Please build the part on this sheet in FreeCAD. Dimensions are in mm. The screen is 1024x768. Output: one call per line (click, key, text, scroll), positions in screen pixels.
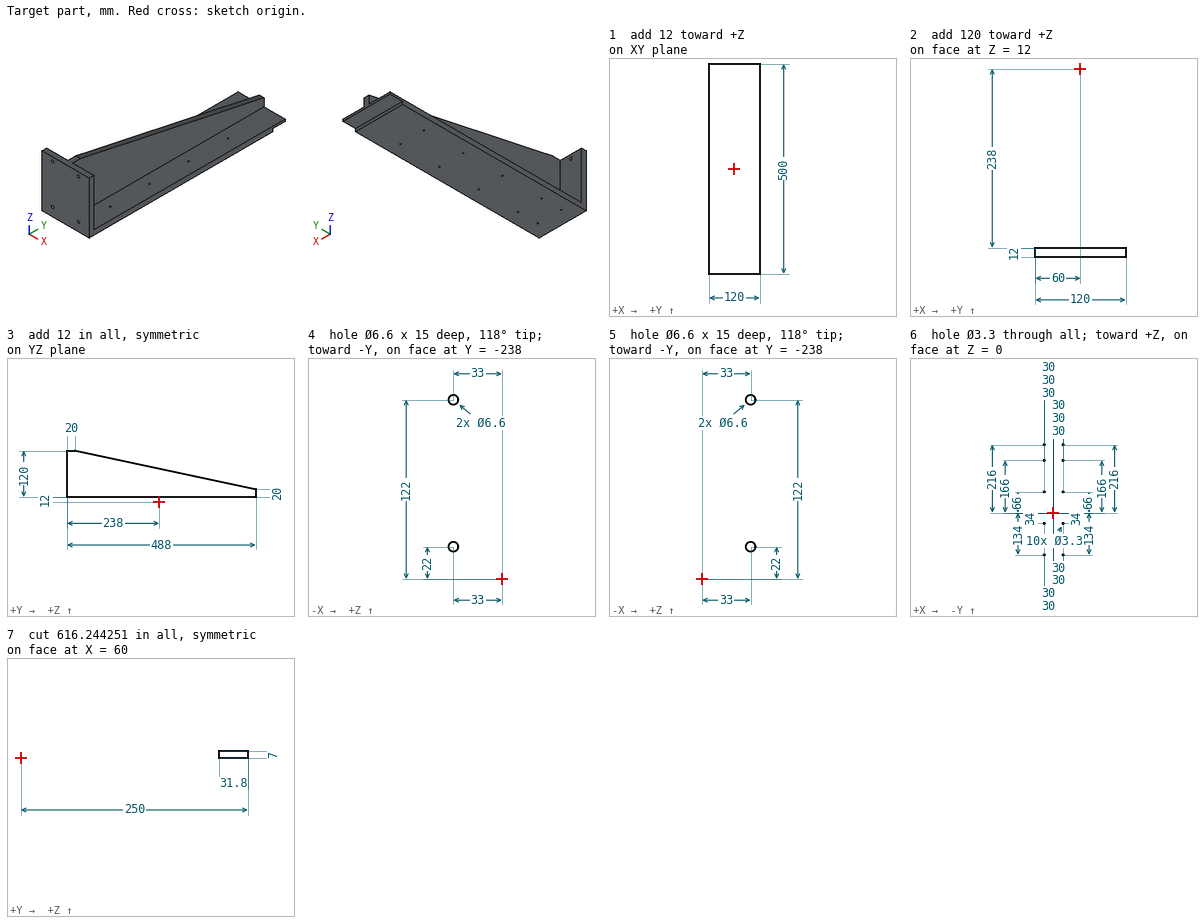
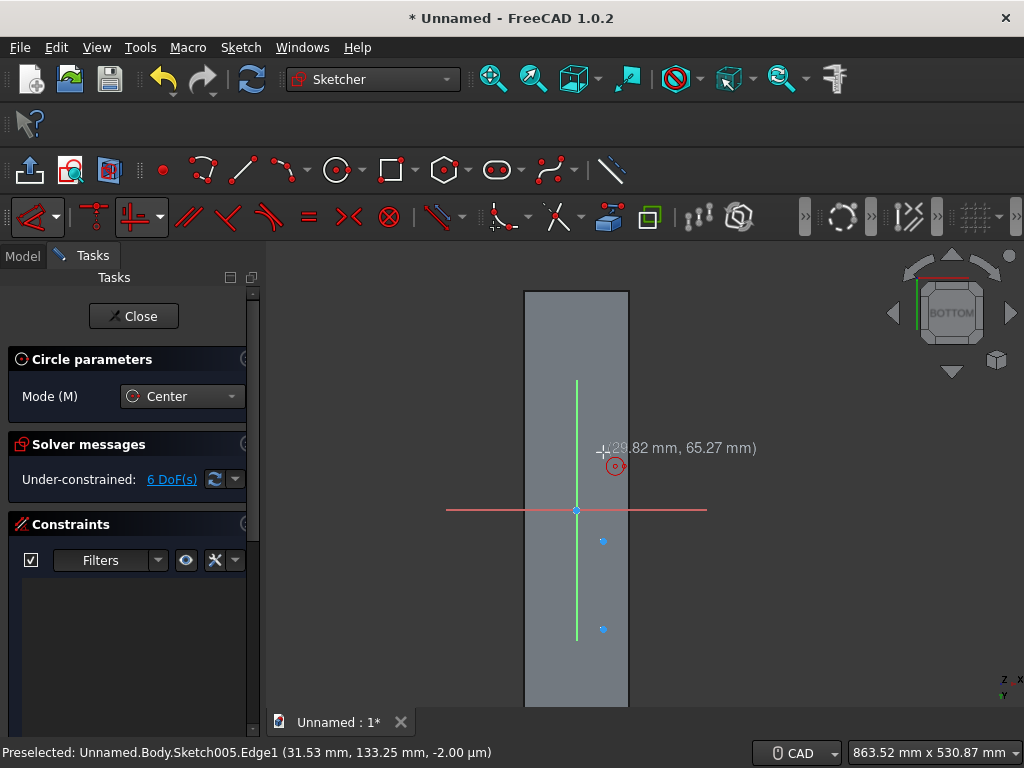
click(603, 452)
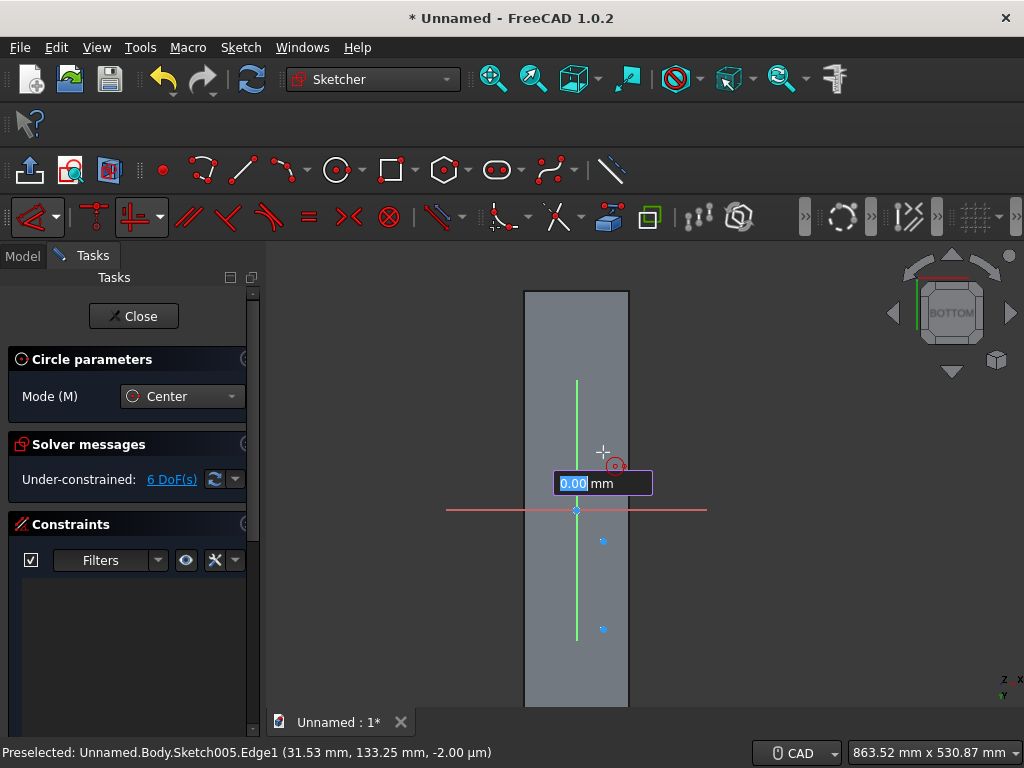
scroll(604, 451, up, 12)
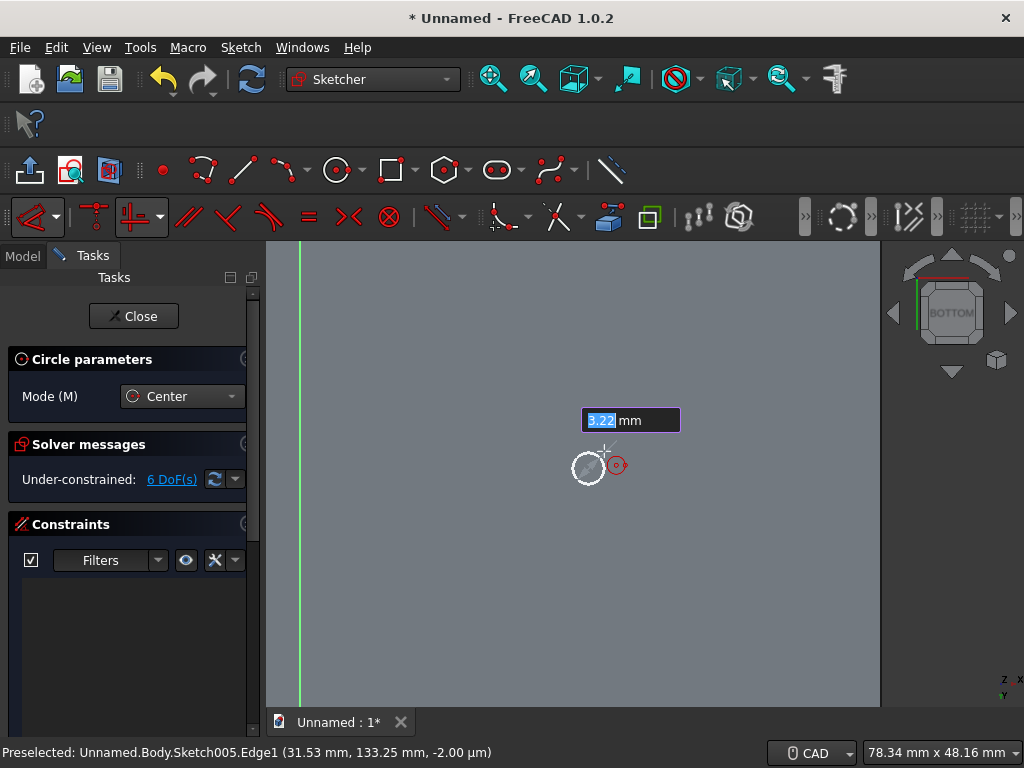
click(602, 450)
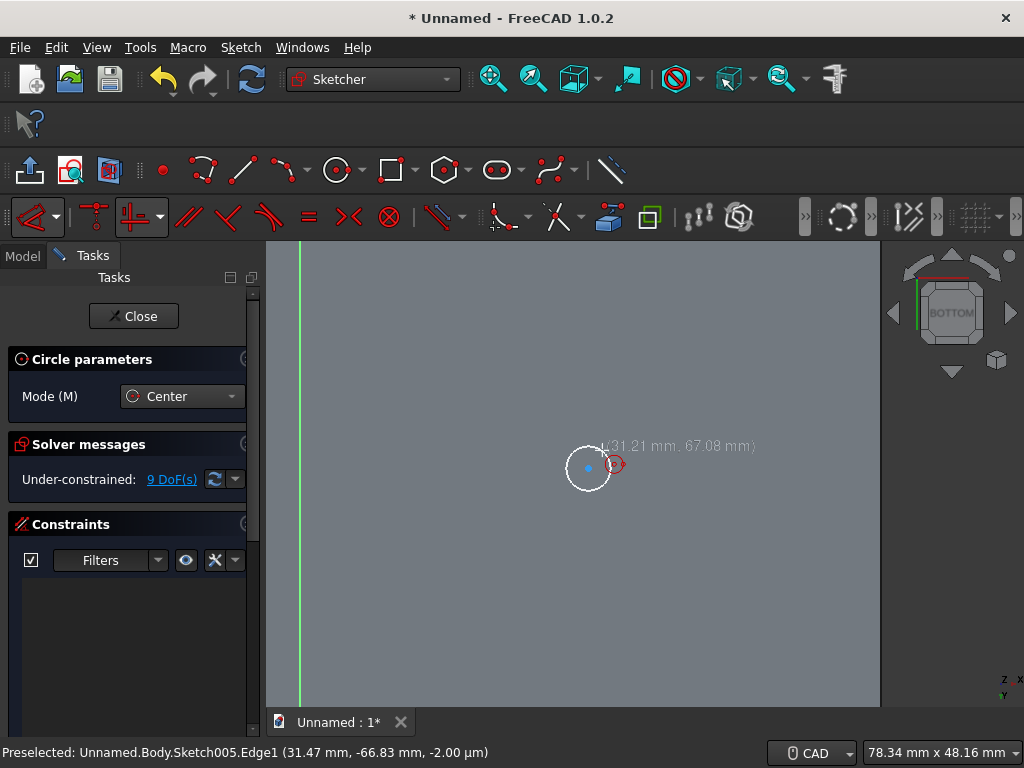
scroll(604, 451, down, 12)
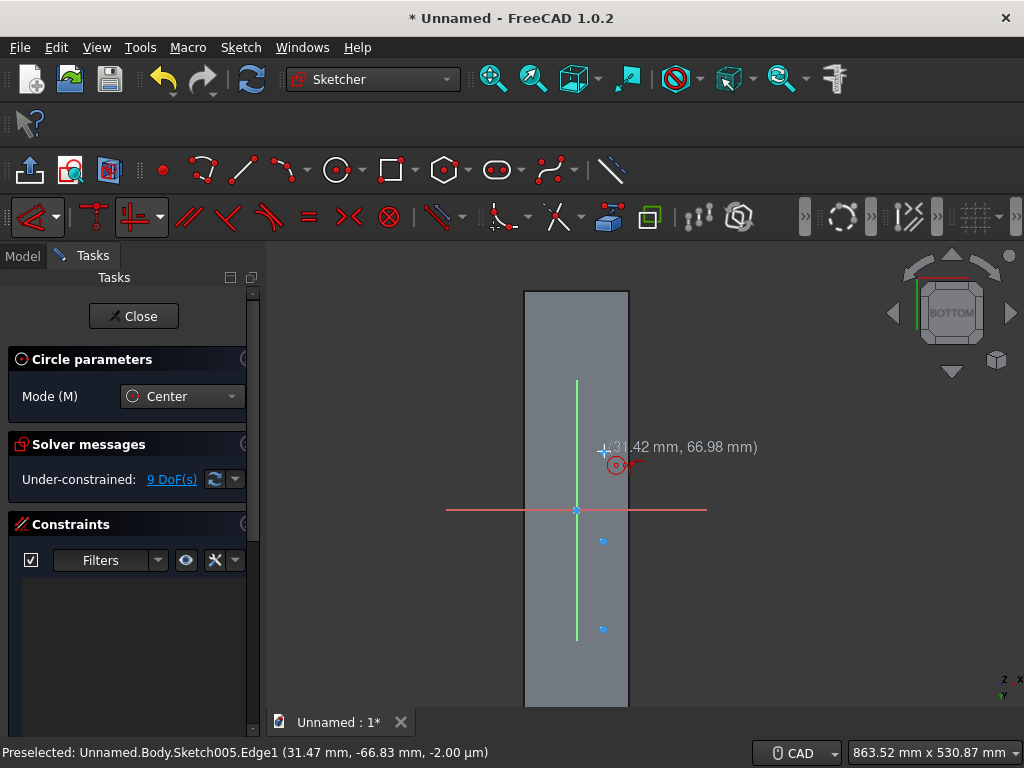
scroll(603, 365, up, 14)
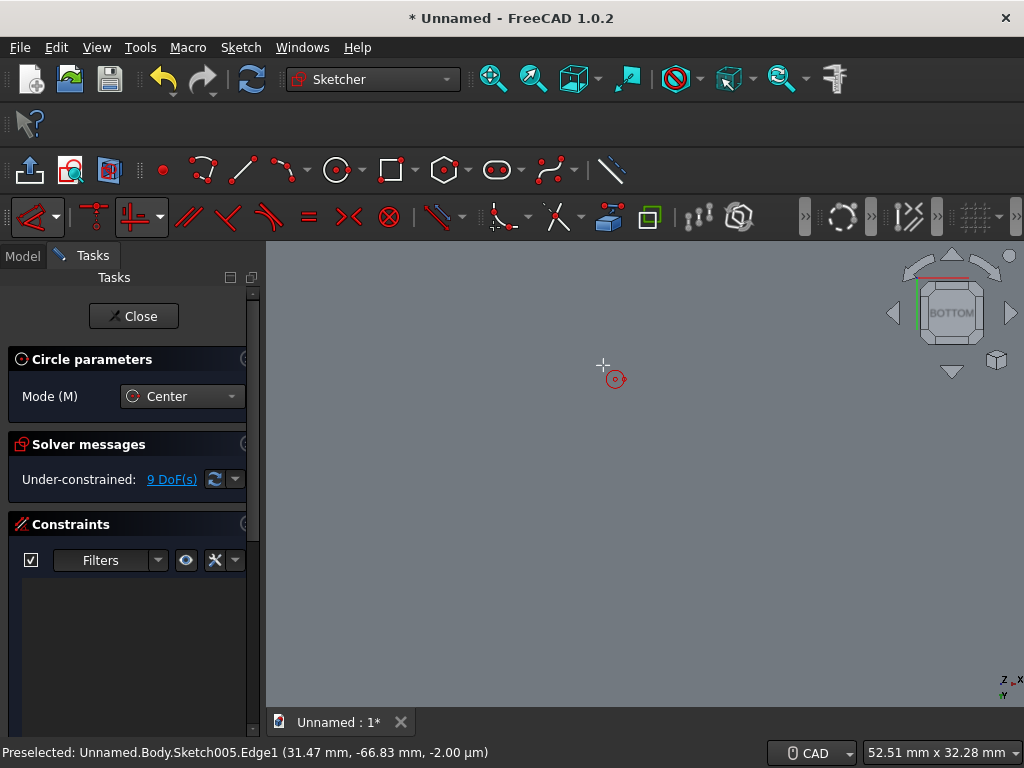
scroll(603, 365, down, 14)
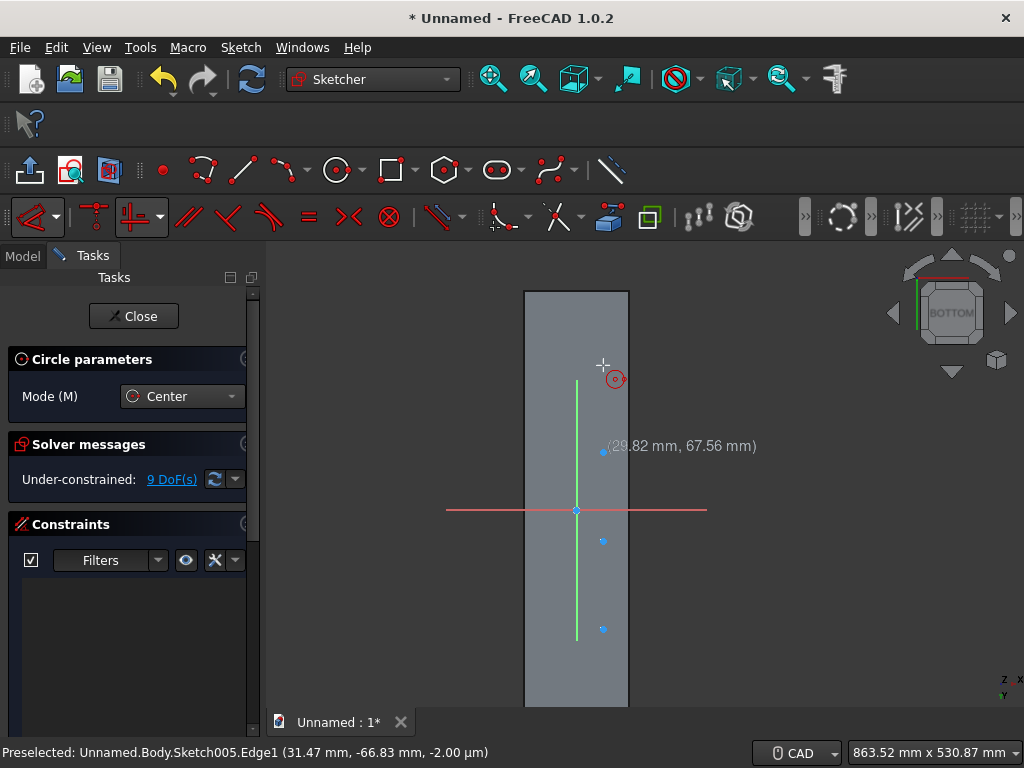
click(603, 365)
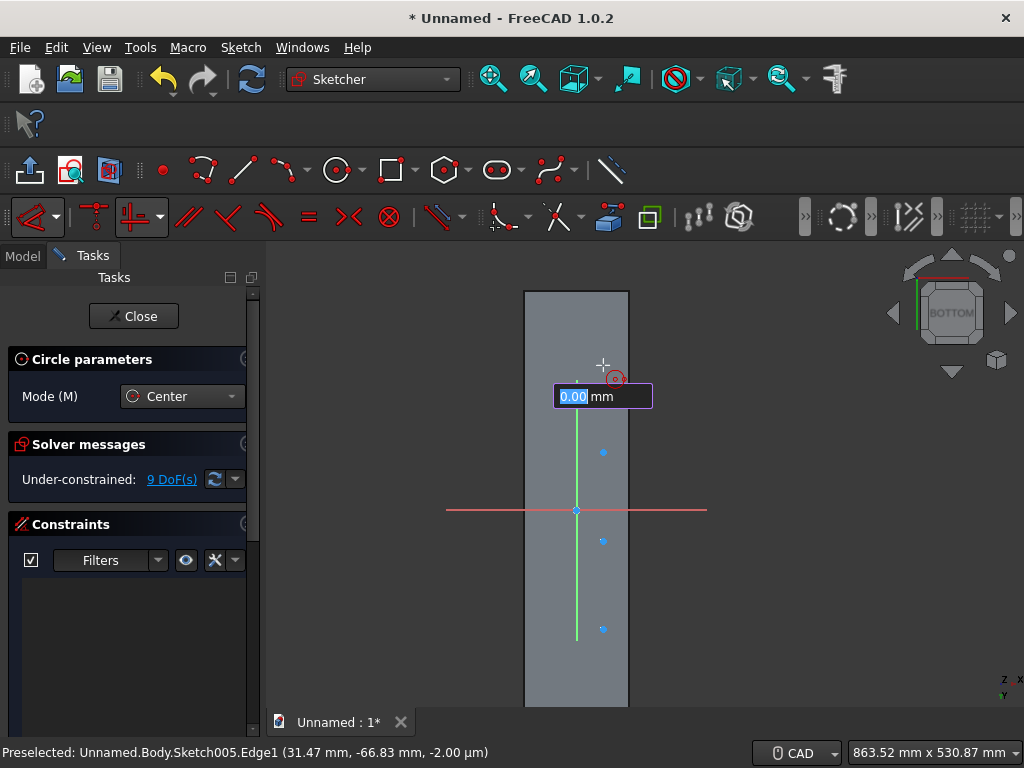
scroll(604, 364, up, 12)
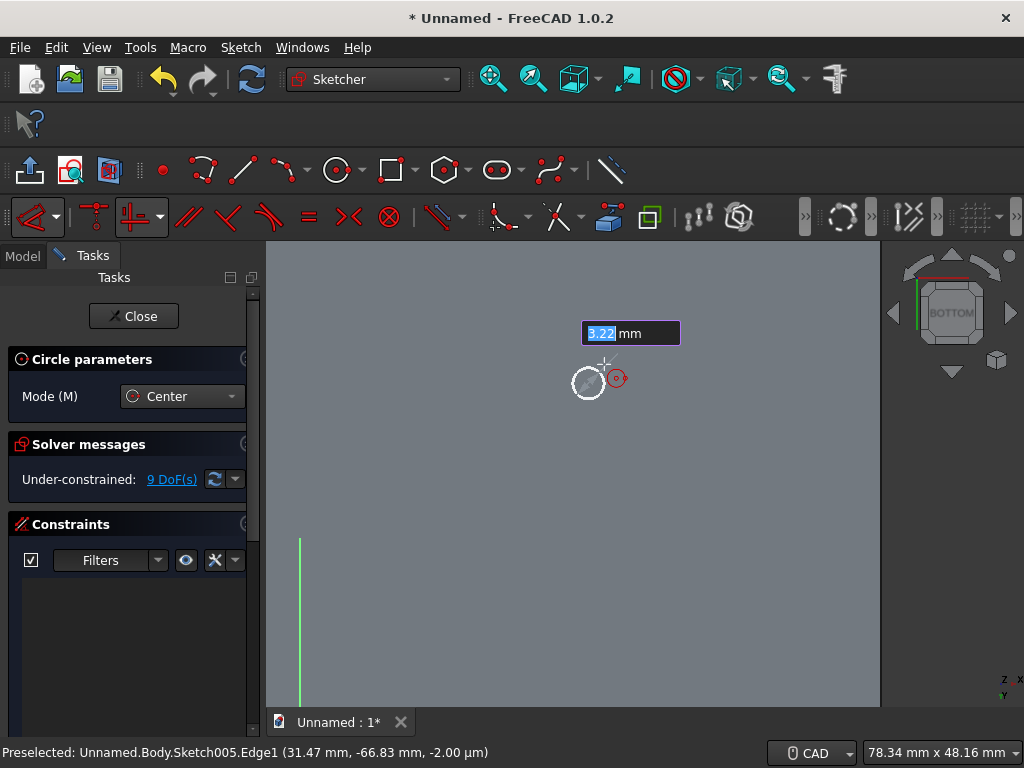
click(602, 356)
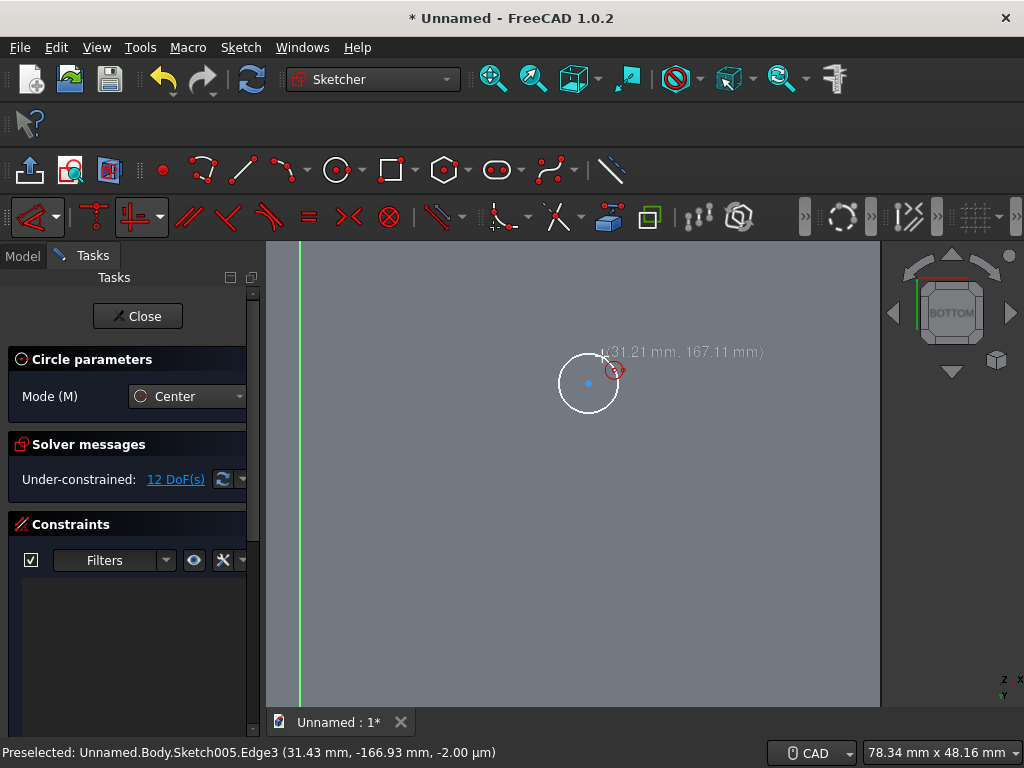
scroll(604, 364, down, 12)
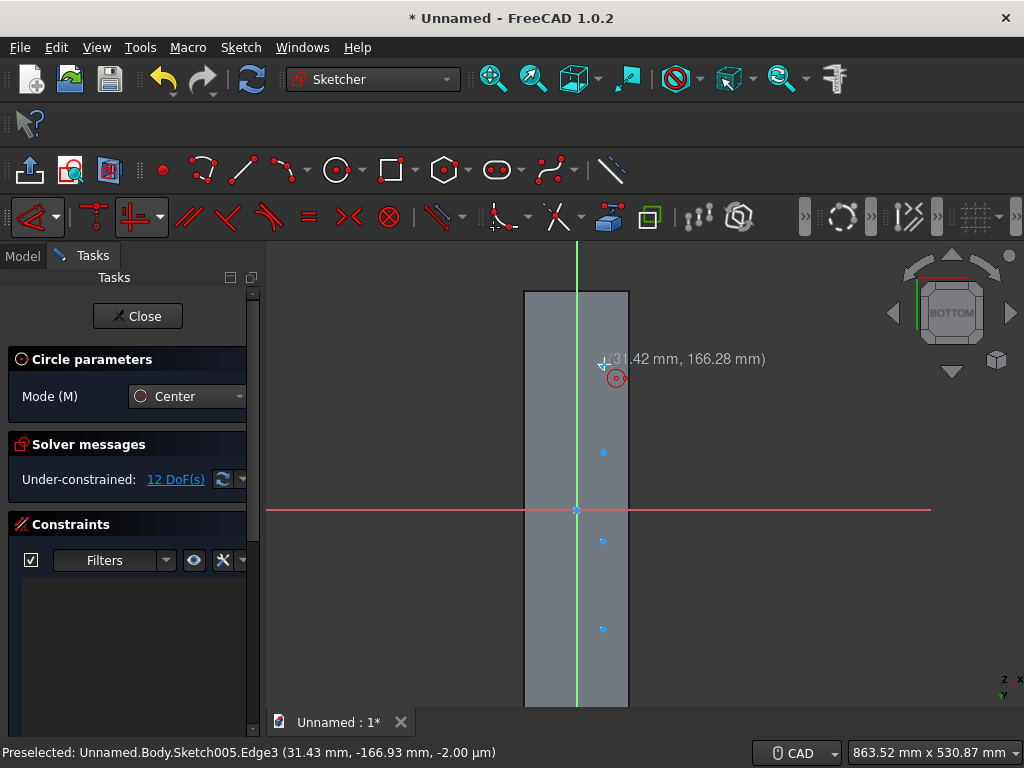
scroll(603, 321, up, 14)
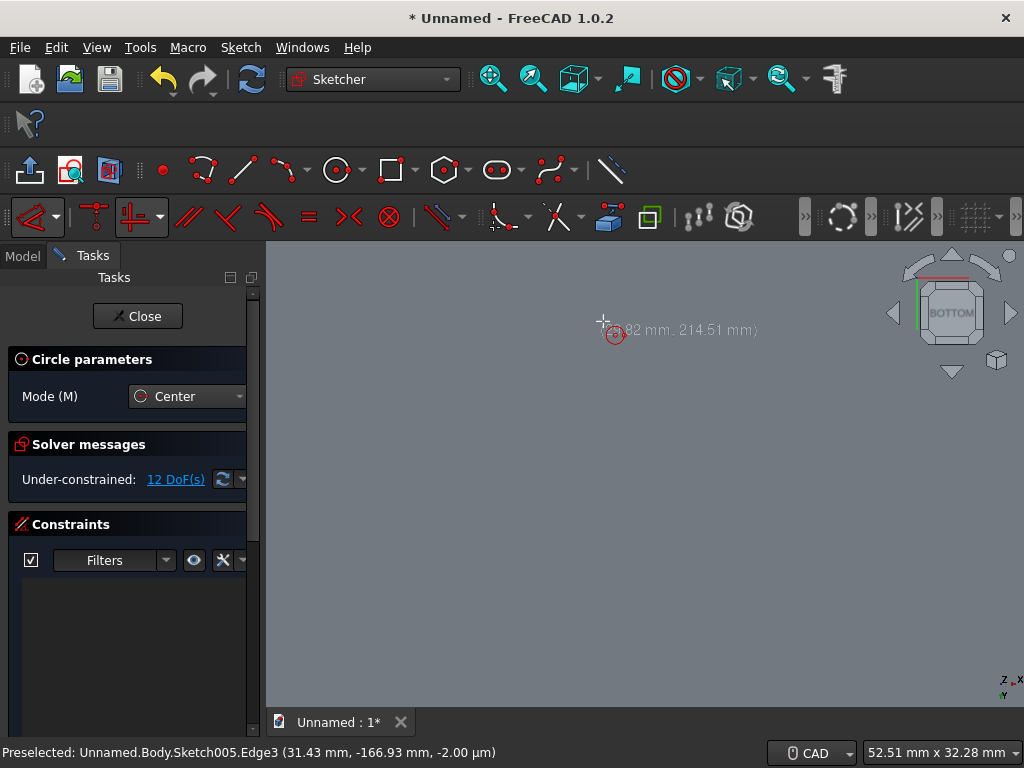
scroll(603, 321, down, 14)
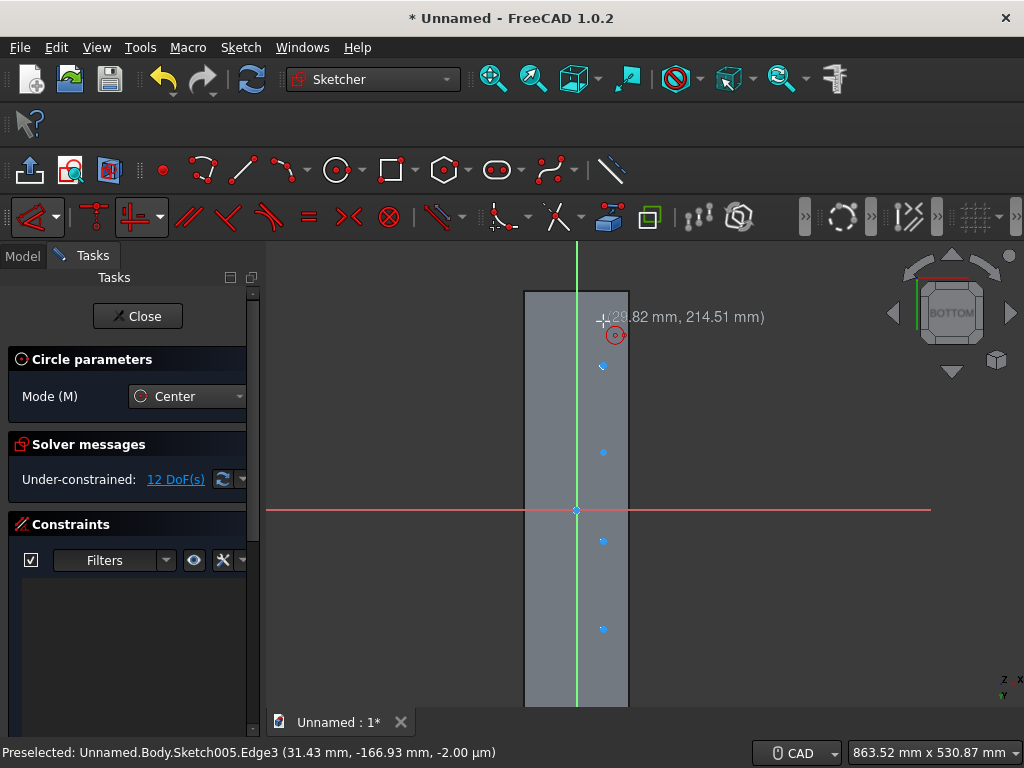
click(603, 321)